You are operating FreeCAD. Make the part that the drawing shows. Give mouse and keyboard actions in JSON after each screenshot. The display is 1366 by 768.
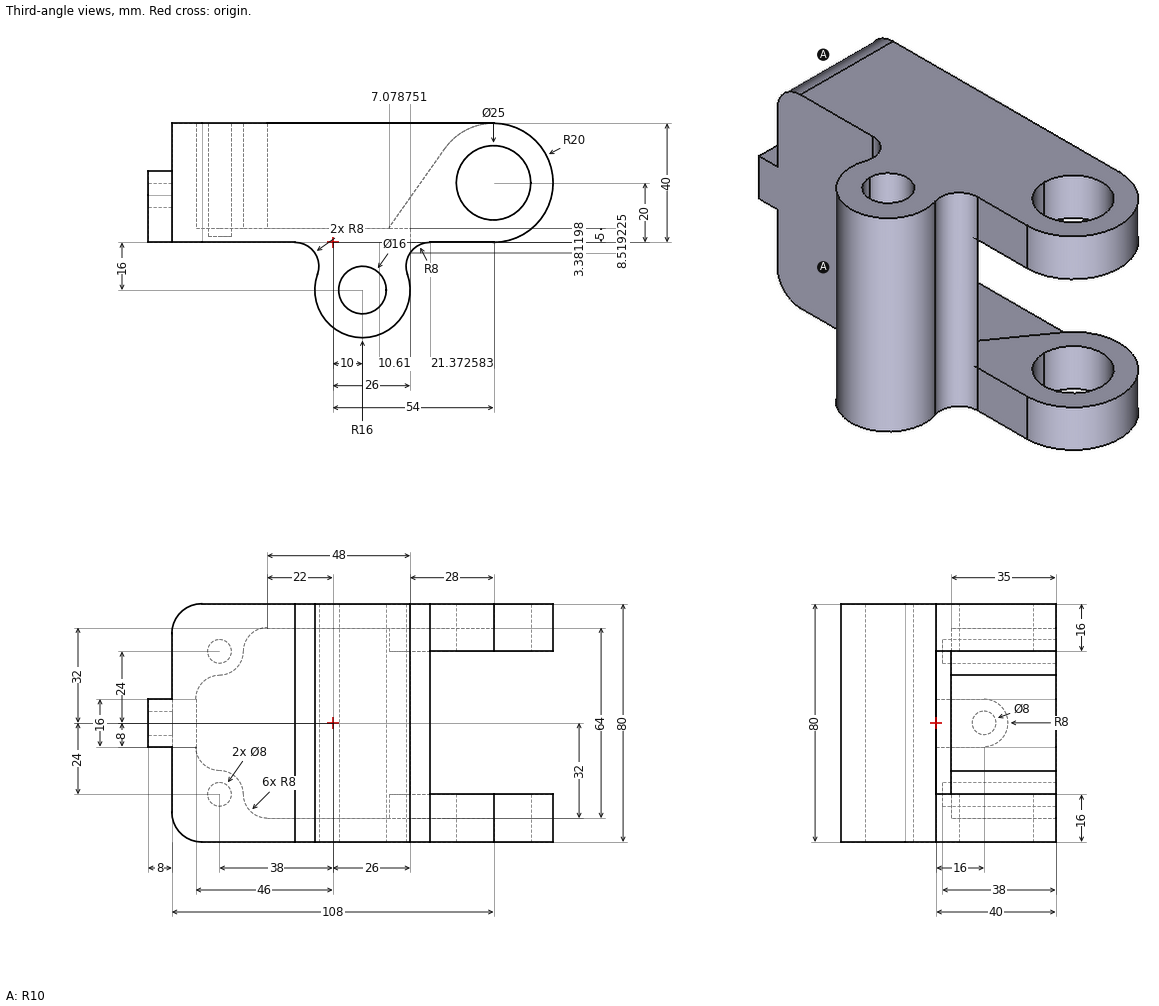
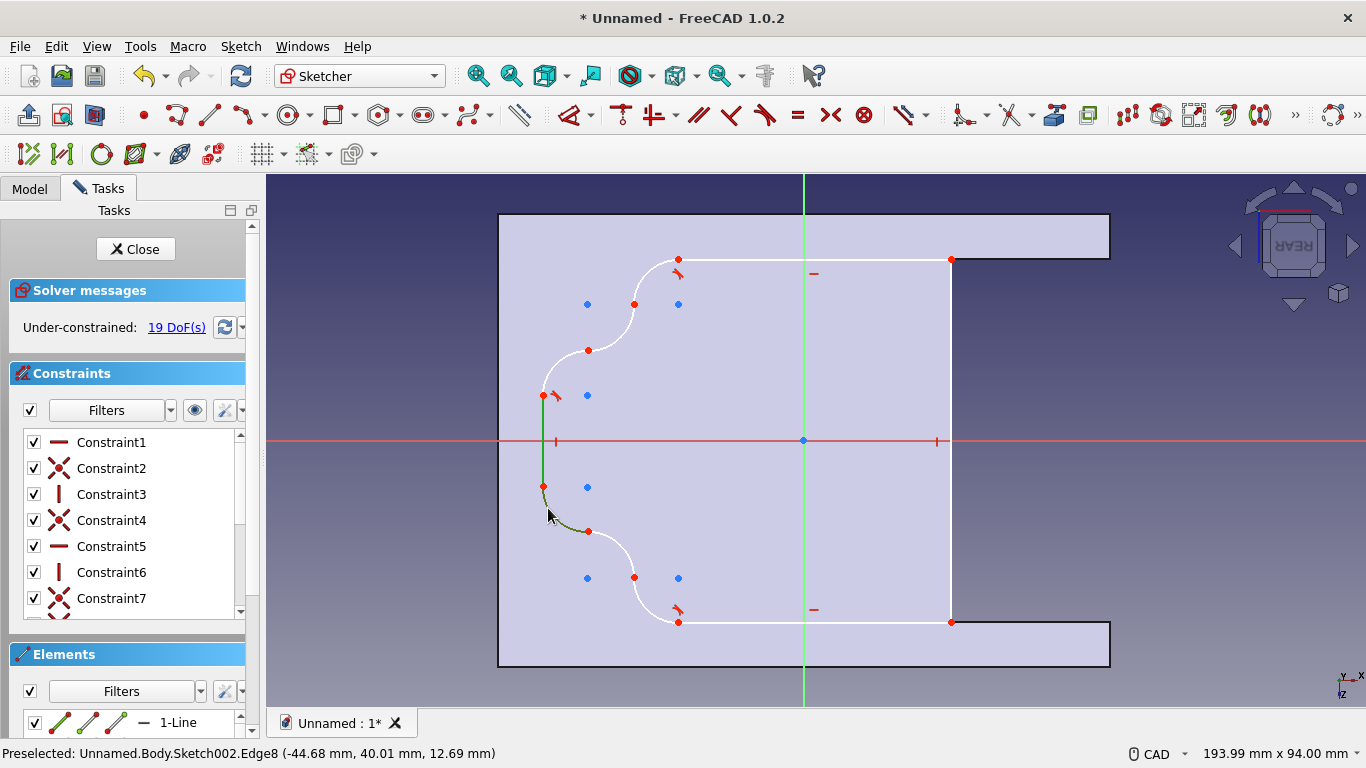
{"action": "key", "text": "t"}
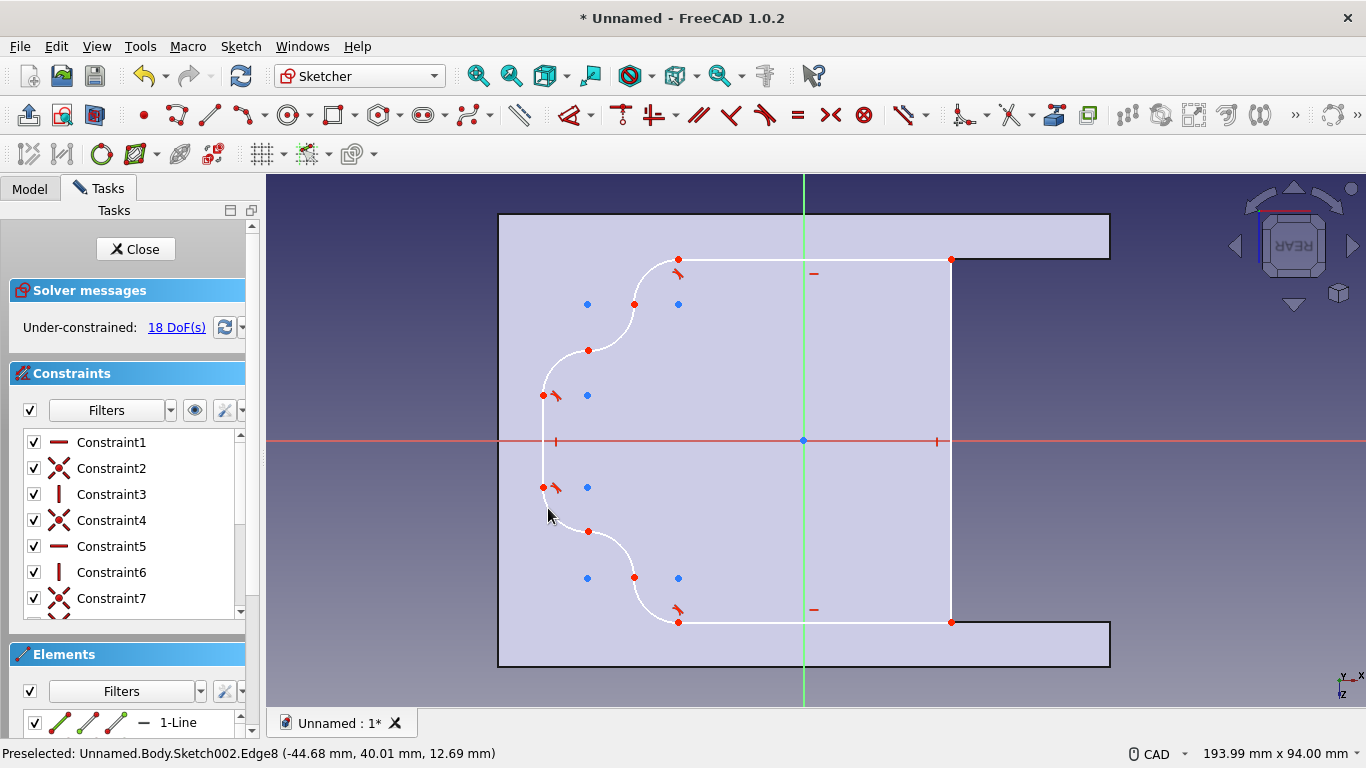
{"action": "left_click", "coordinate": [659, 265]}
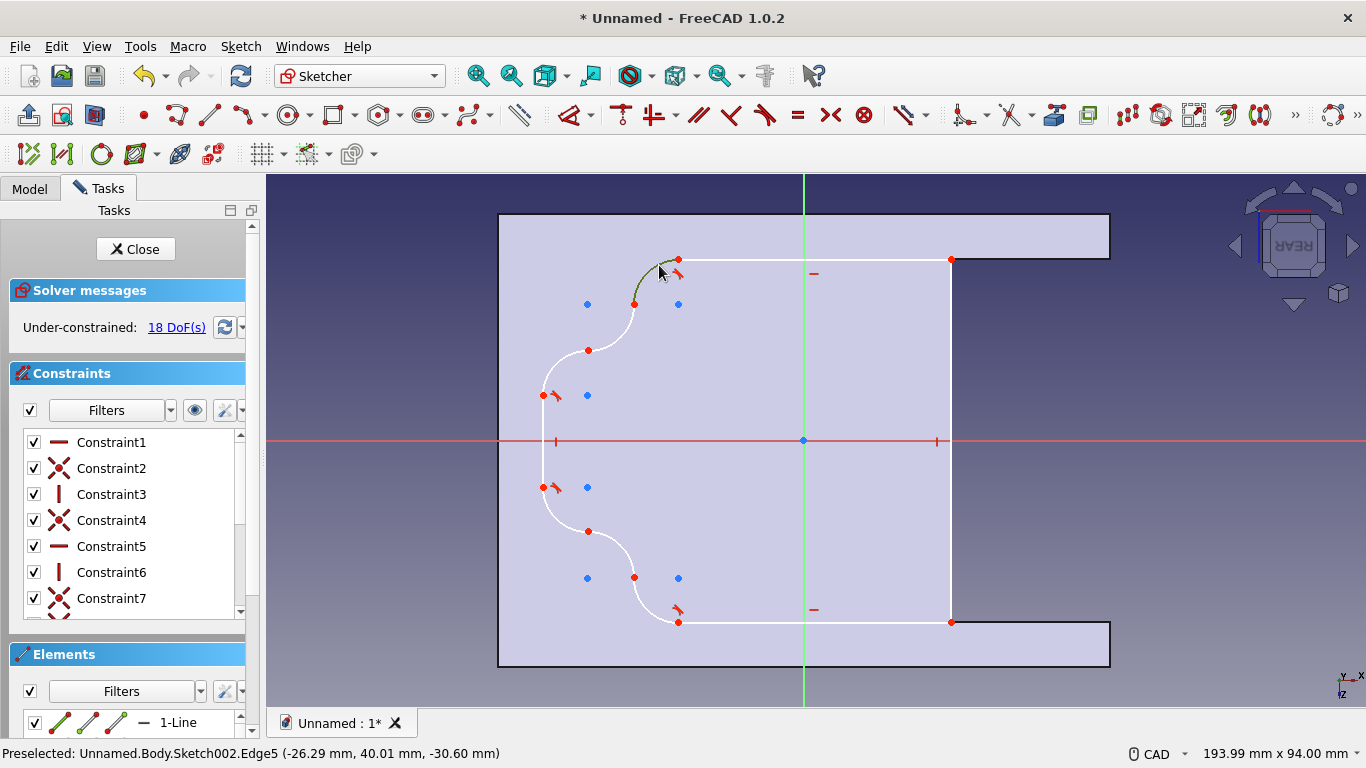
{"action": "left_click", "coordinate": [609, 346]}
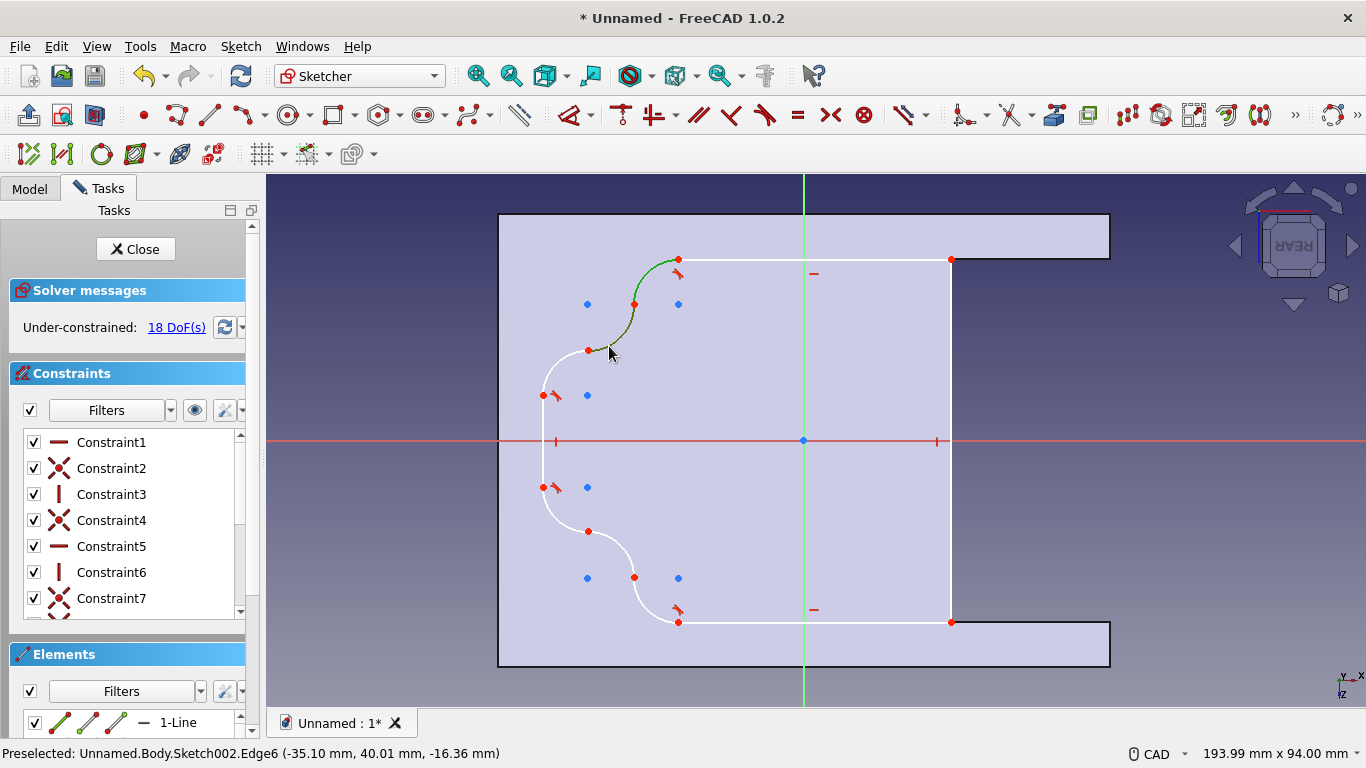
{"action": "key", "text": "t"}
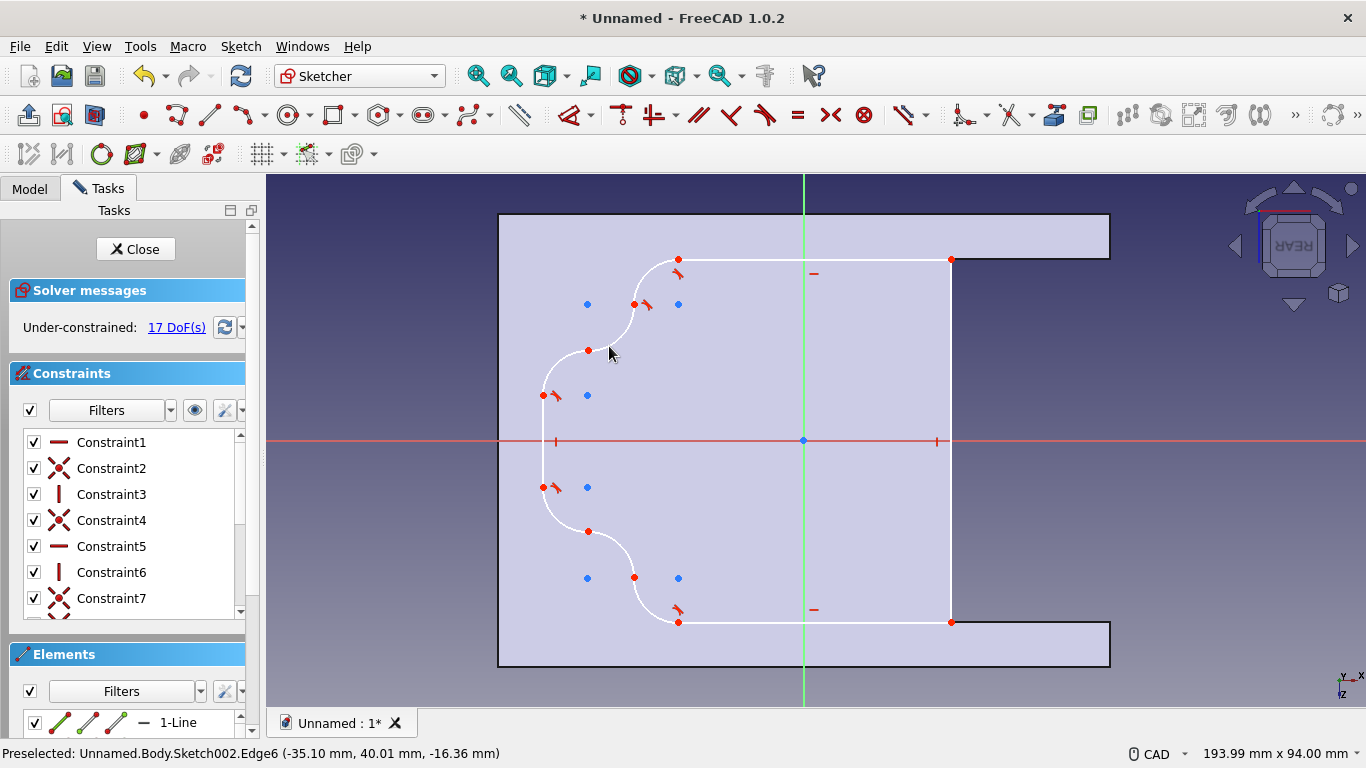
{"action": "left_click", "coordinate": [609, 346]}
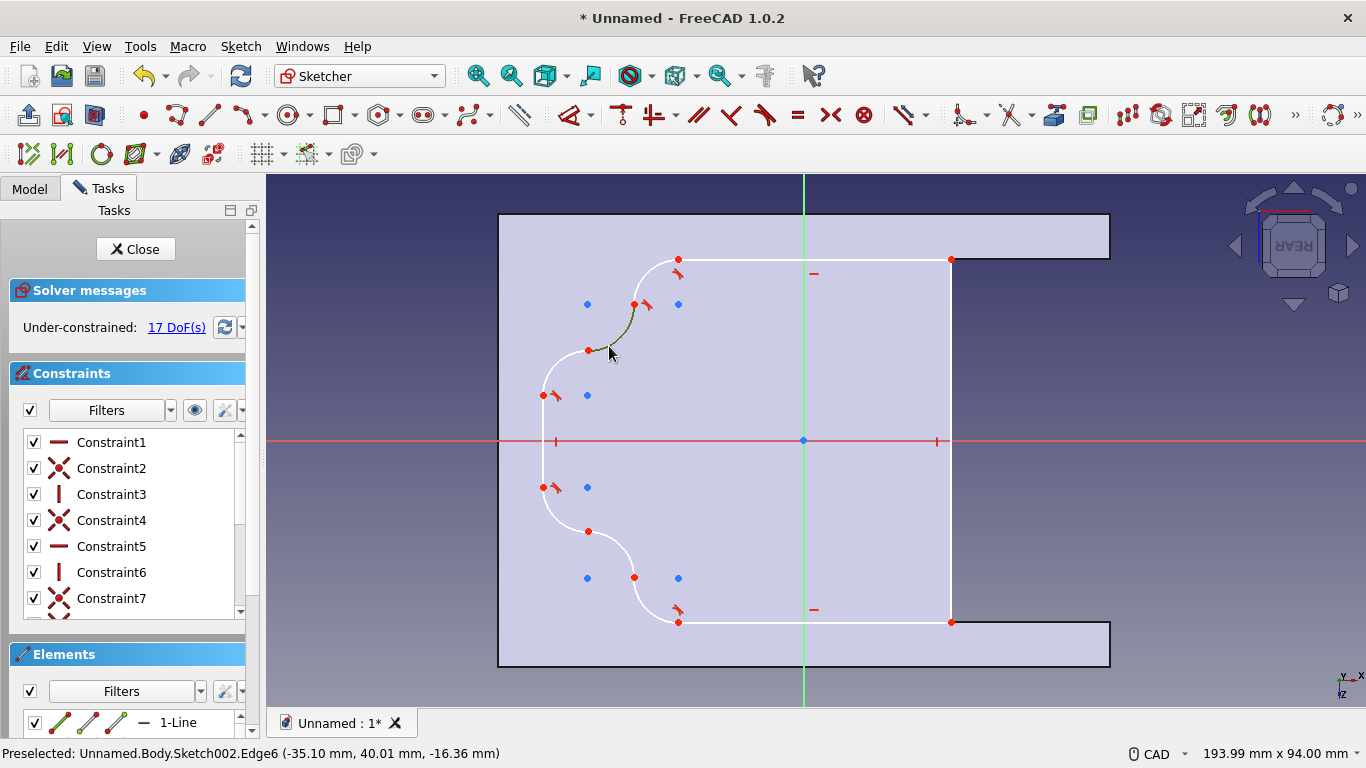
{"action": "left_click", "coordinate": [568, 356]}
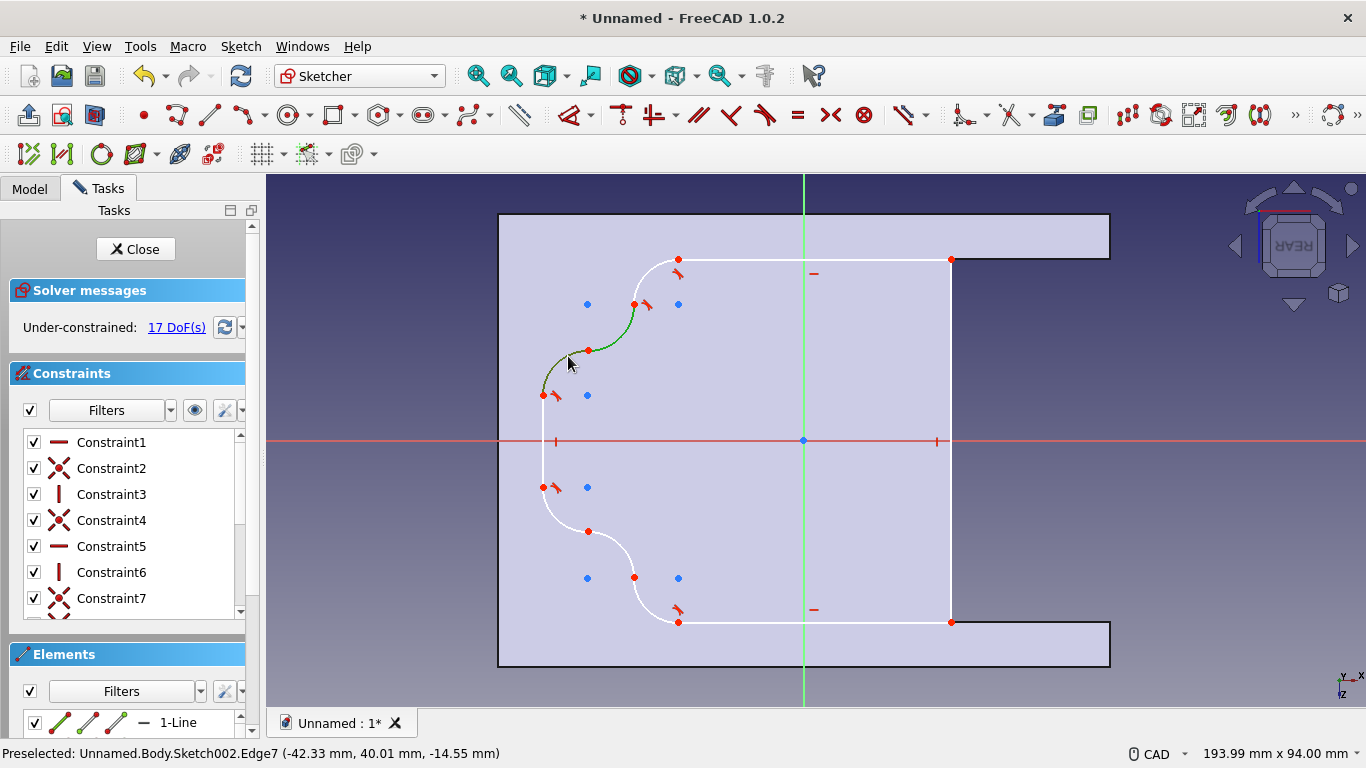
{"action": "left_click", "coordinate": [765, 116]}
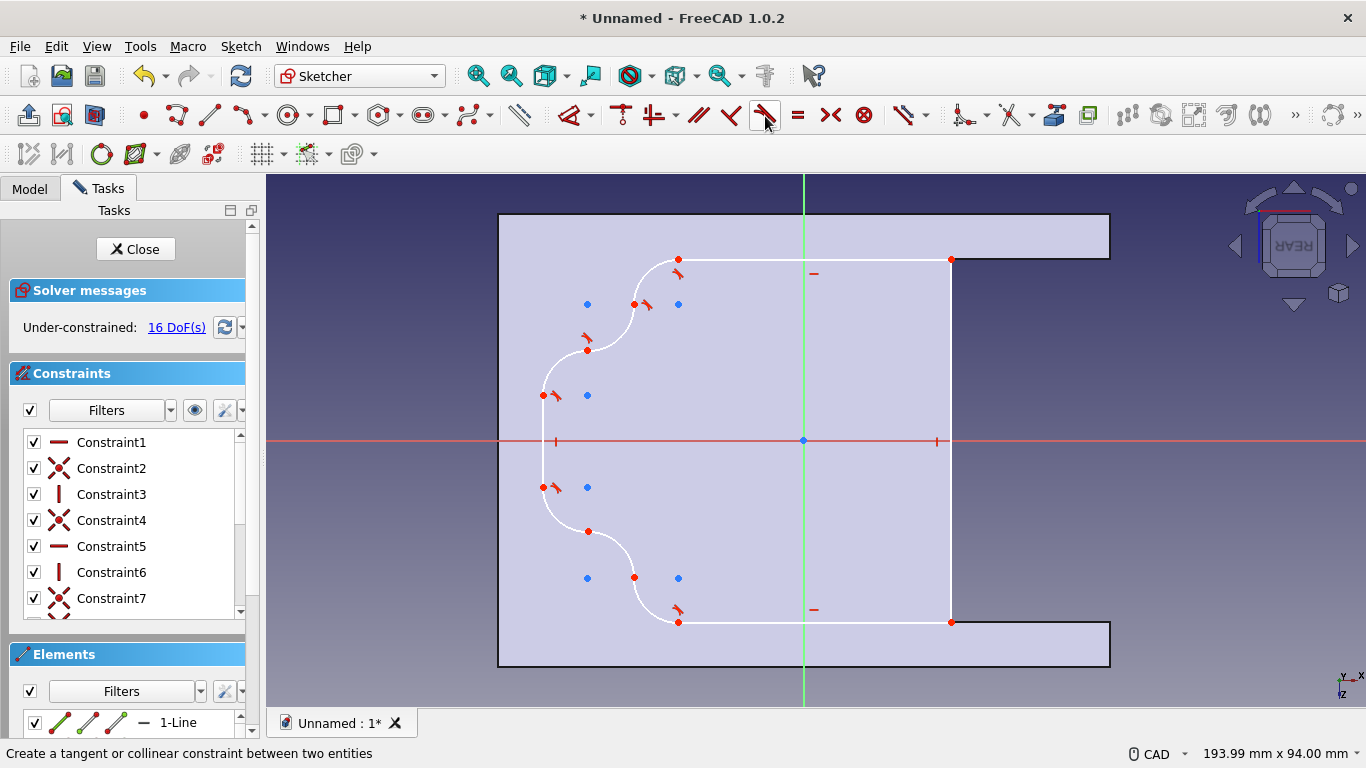
{"action": "left_click", "coordinate": [548, 507]}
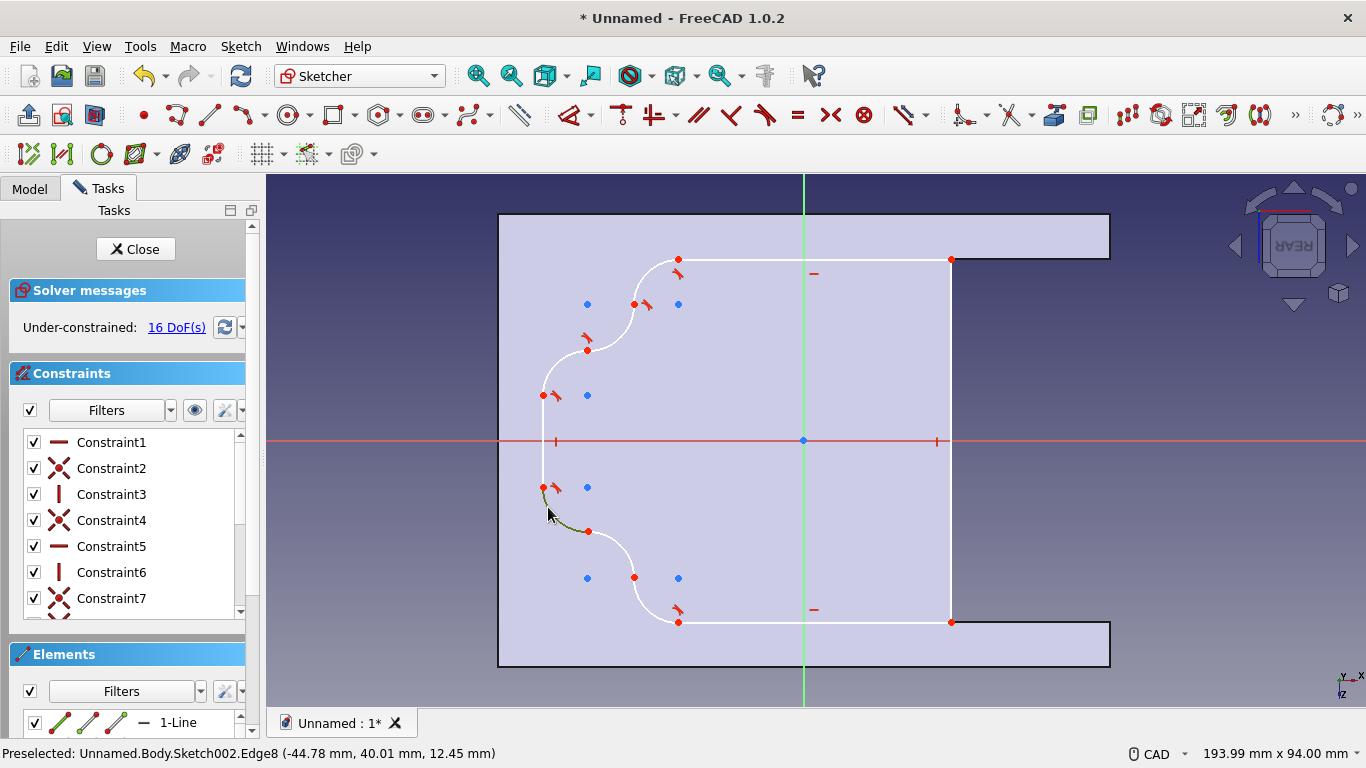
{"action": "left_click", "coordinate": [629, 557]}